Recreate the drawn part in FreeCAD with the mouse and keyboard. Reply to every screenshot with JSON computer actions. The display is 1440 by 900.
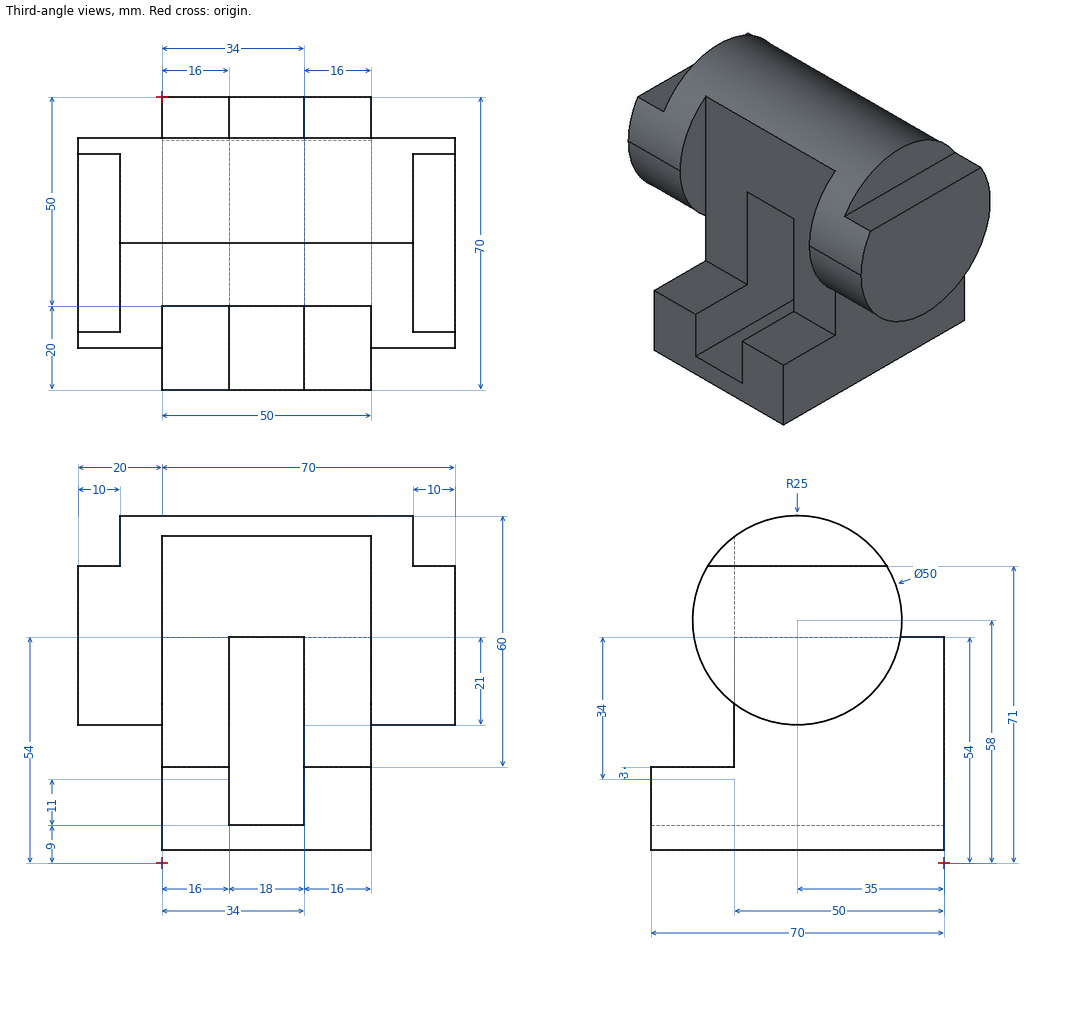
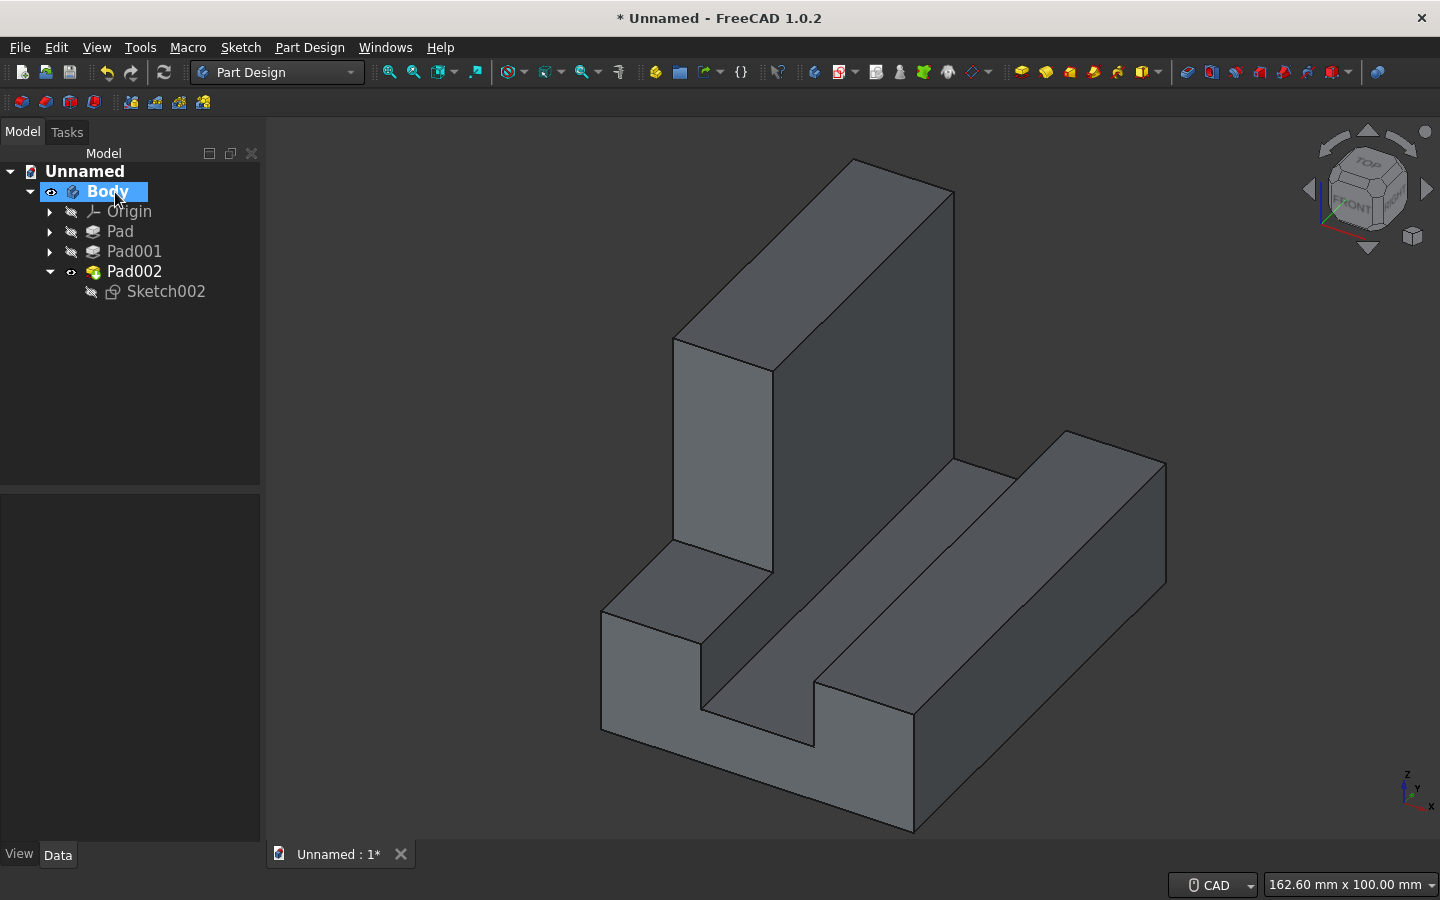
{"action": "left_click", "coordinate": [968, 719]}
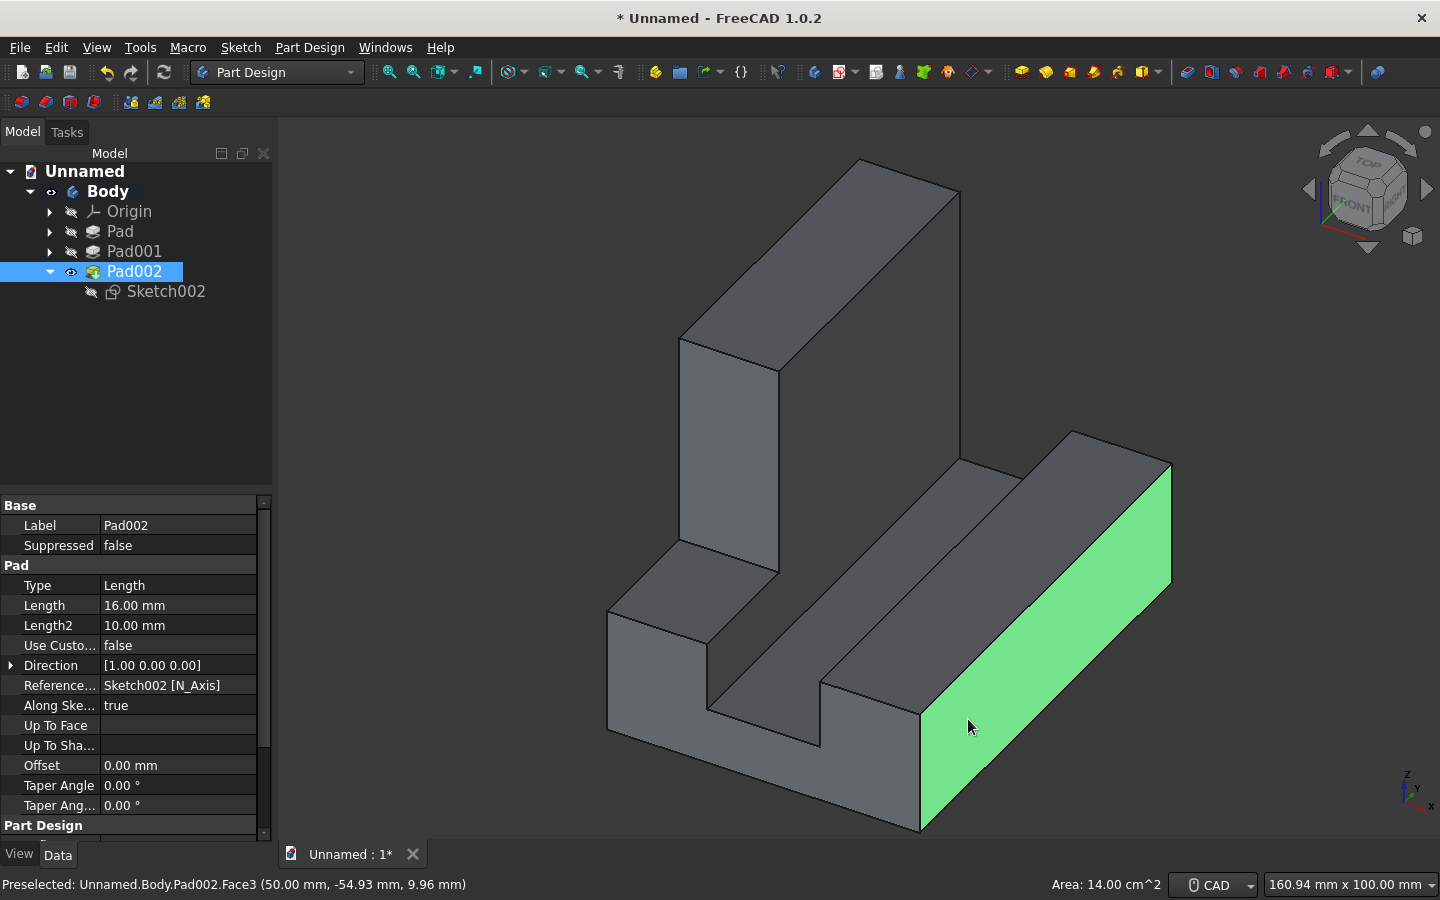
{"action": "left_click", "coordinate": [840, 72]}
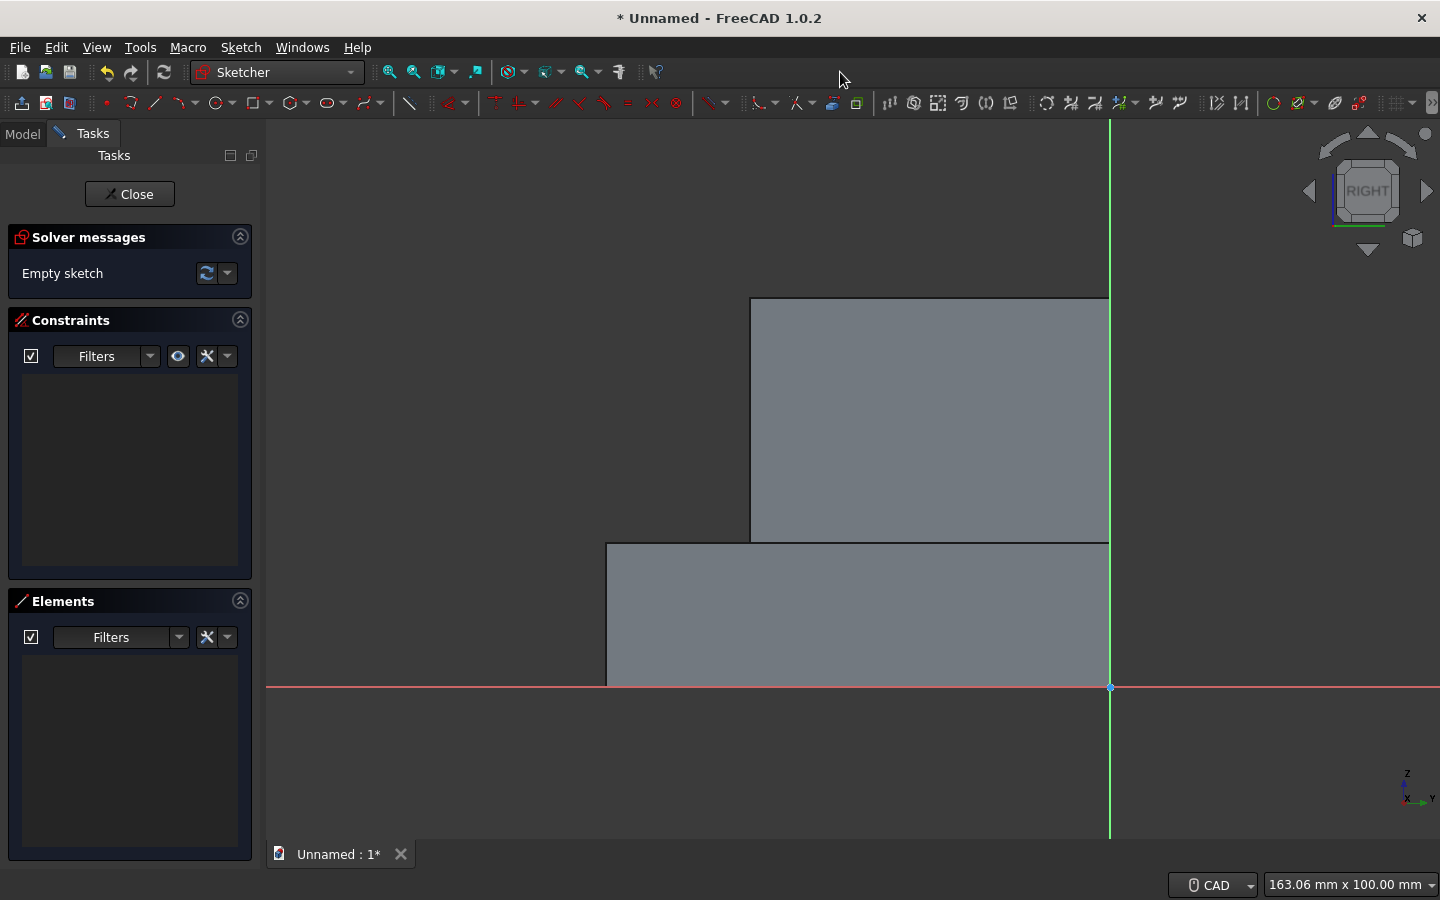
{"action": "left_click", "coordinate": [254, 104]}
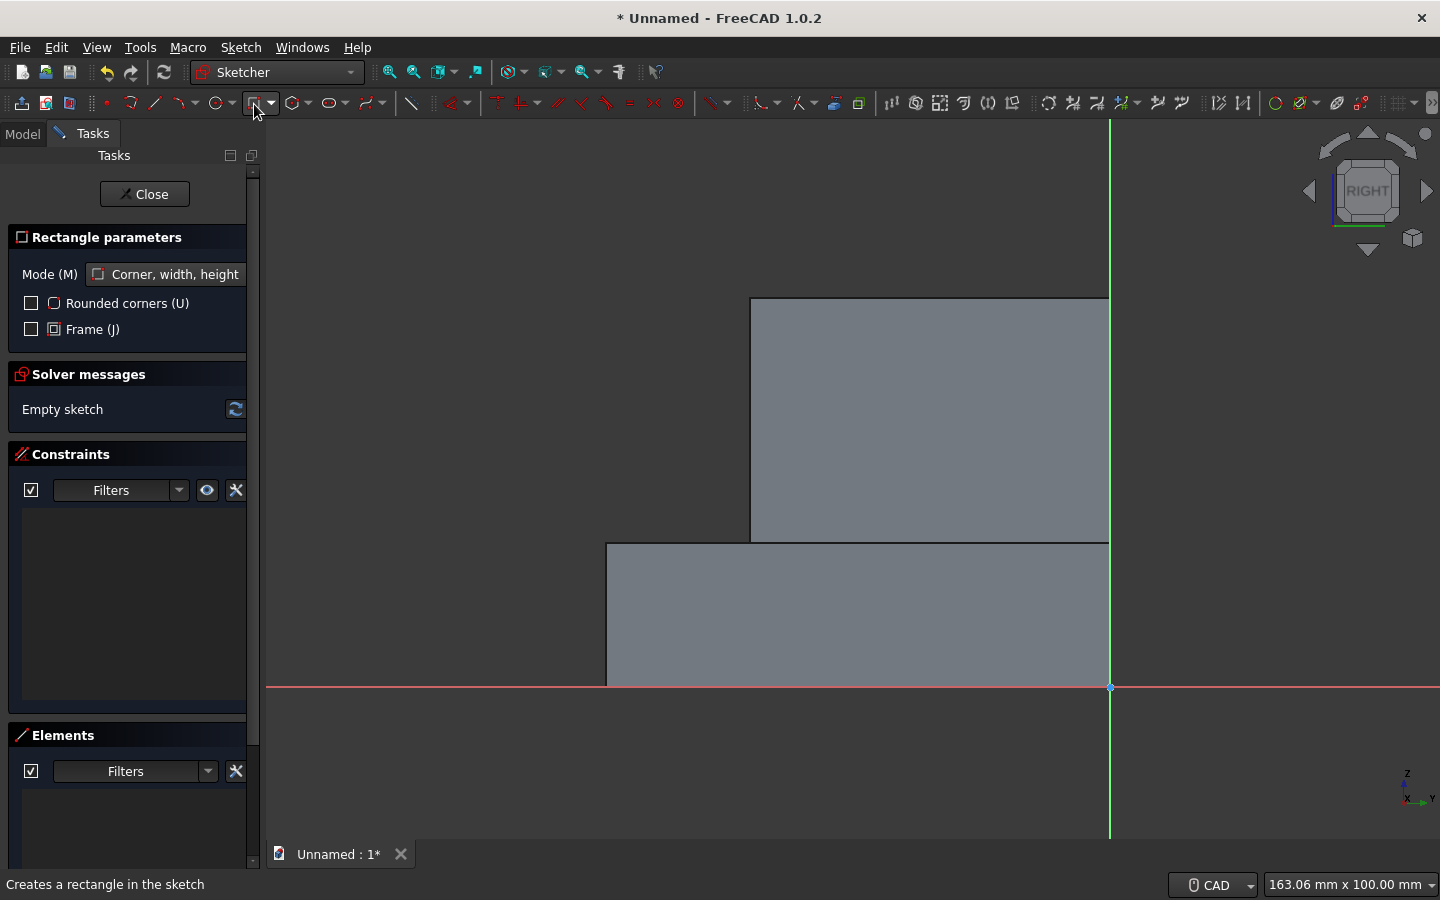
{"action": "left_click", "coordinate": [750, 298]}
{"action": "left_click", "coordinate": [1110, 543]}
{"action": "key", "text": "Escape"}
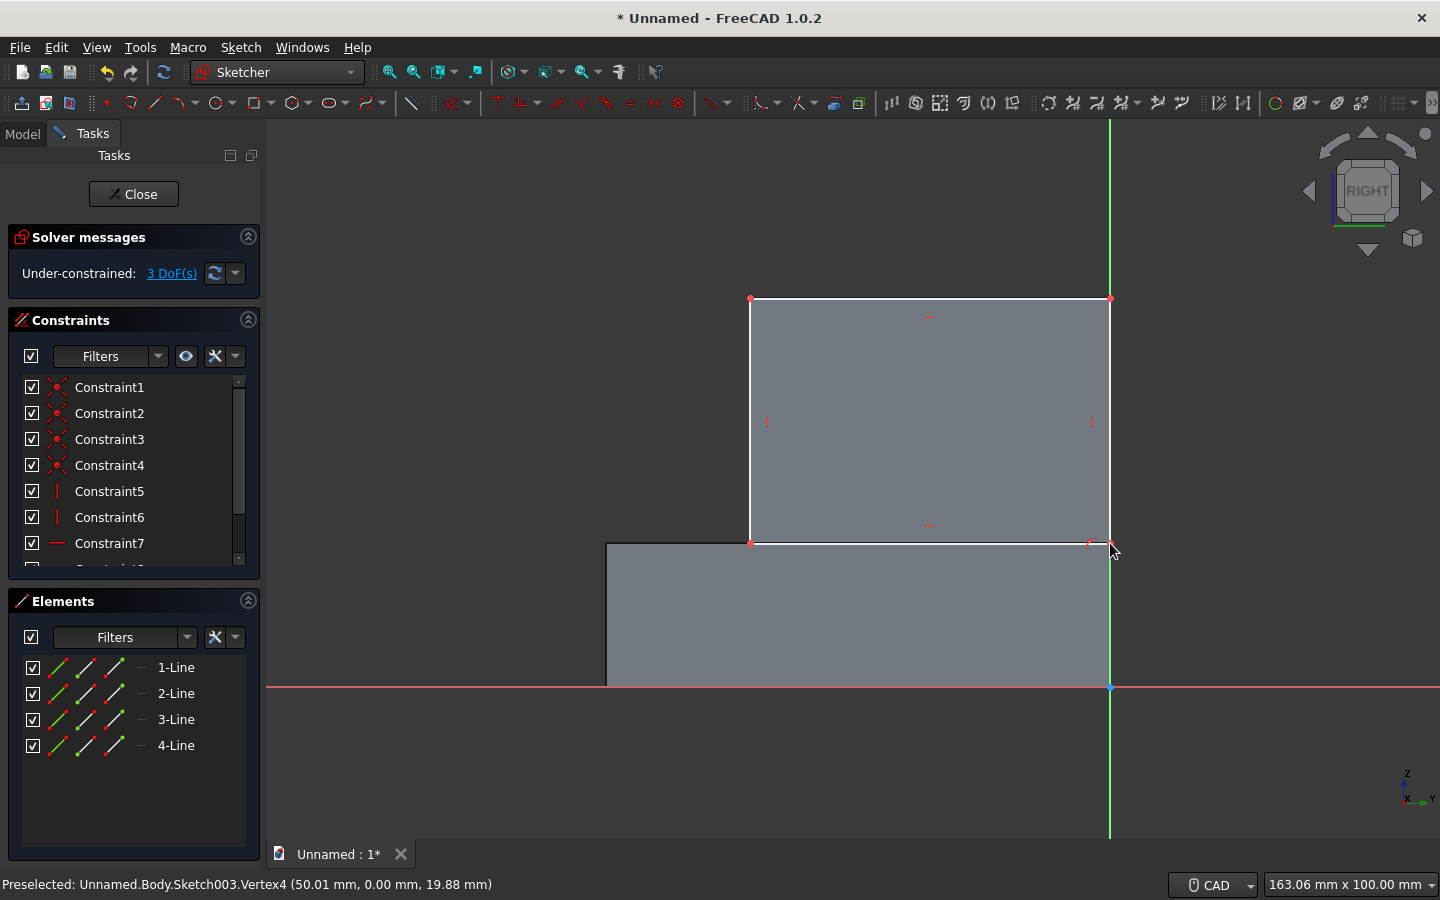
{"action": "left_click", "coordinate": [750, 373]}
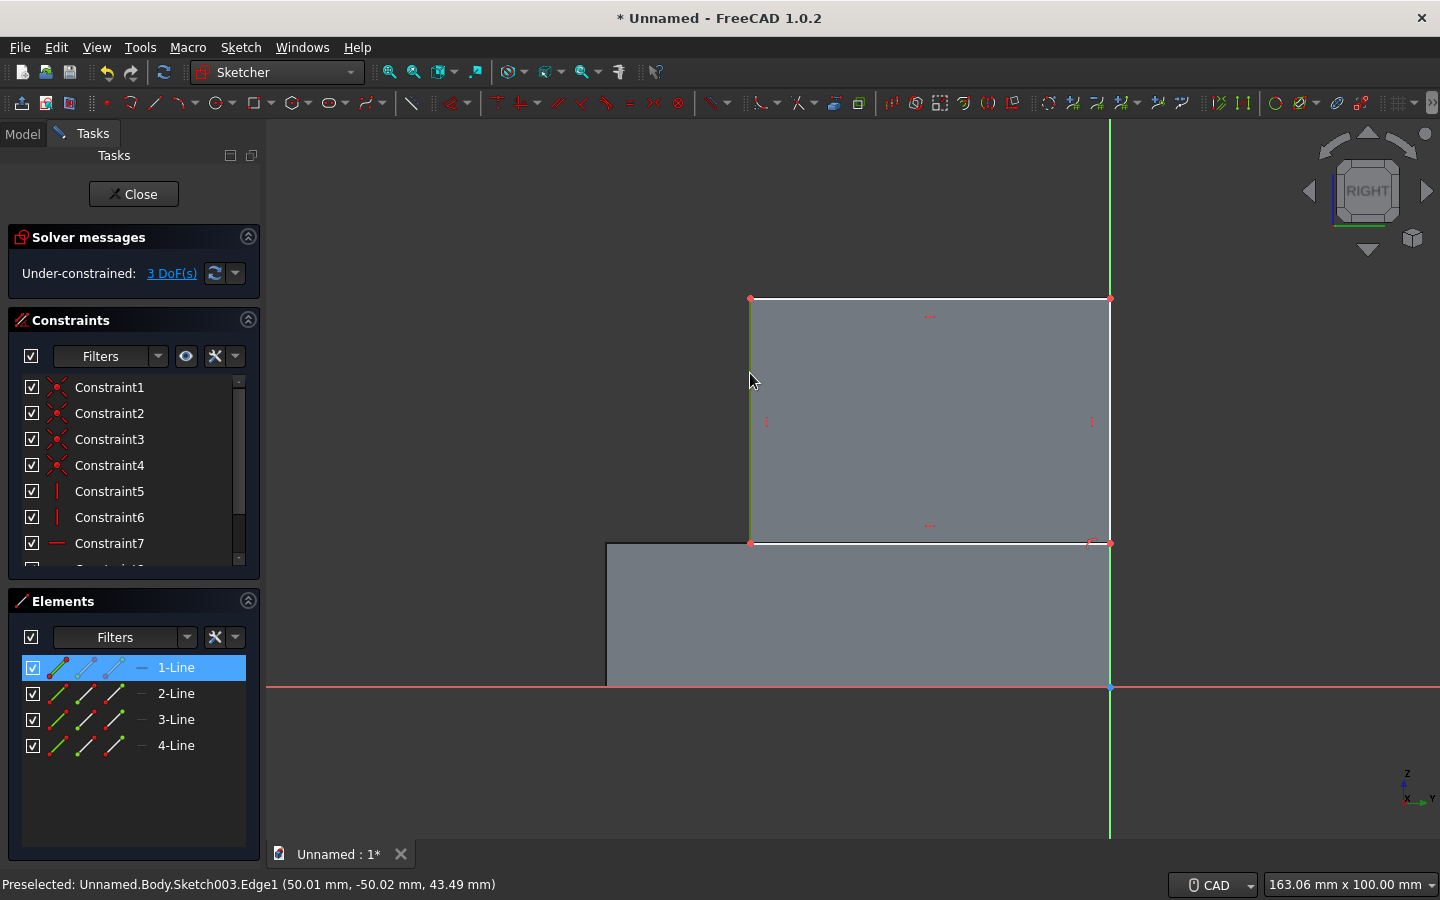
{"action": "left_click", "coordinate": [470, 104]}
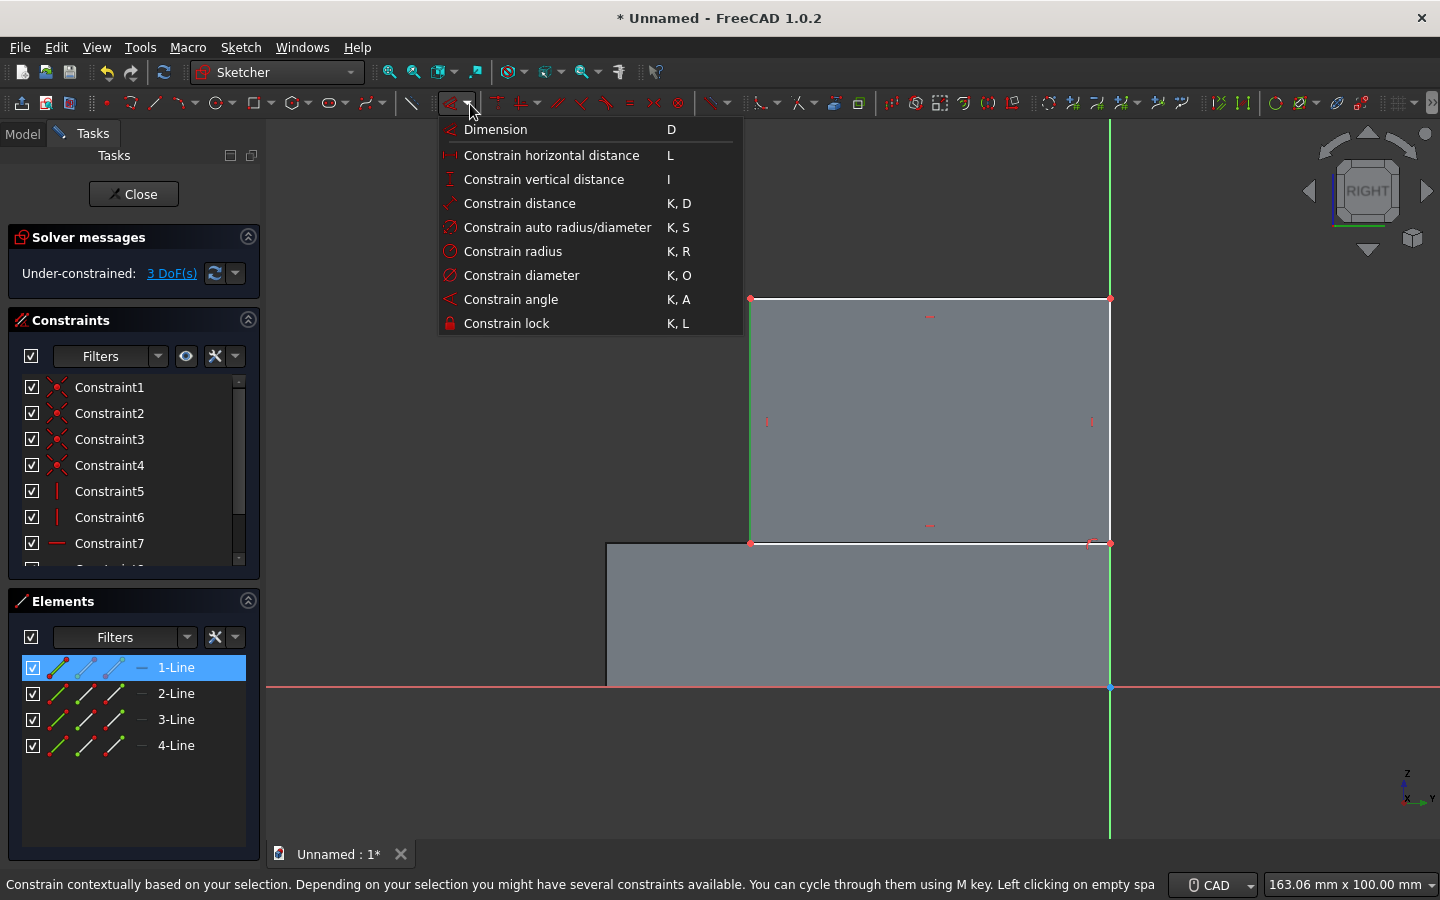
{"action": "left_click", "coordinate": [591, 179]}